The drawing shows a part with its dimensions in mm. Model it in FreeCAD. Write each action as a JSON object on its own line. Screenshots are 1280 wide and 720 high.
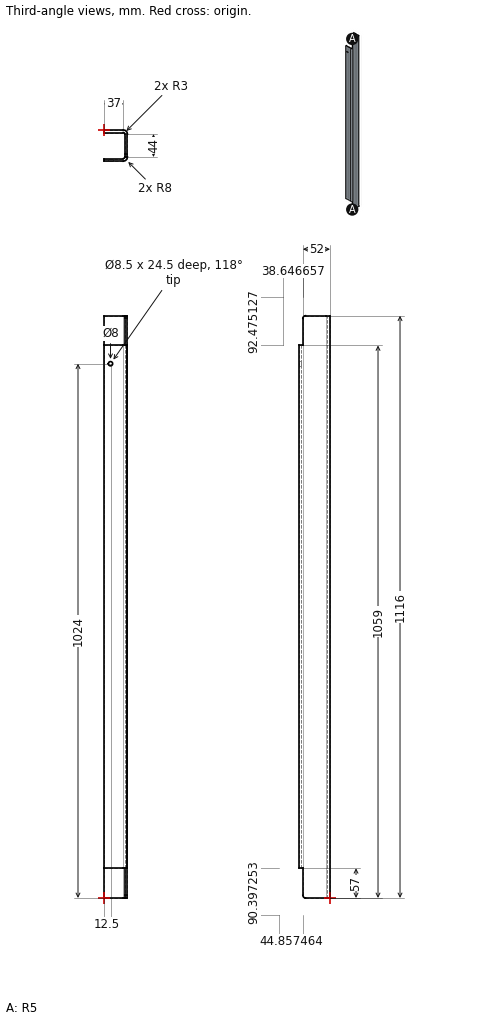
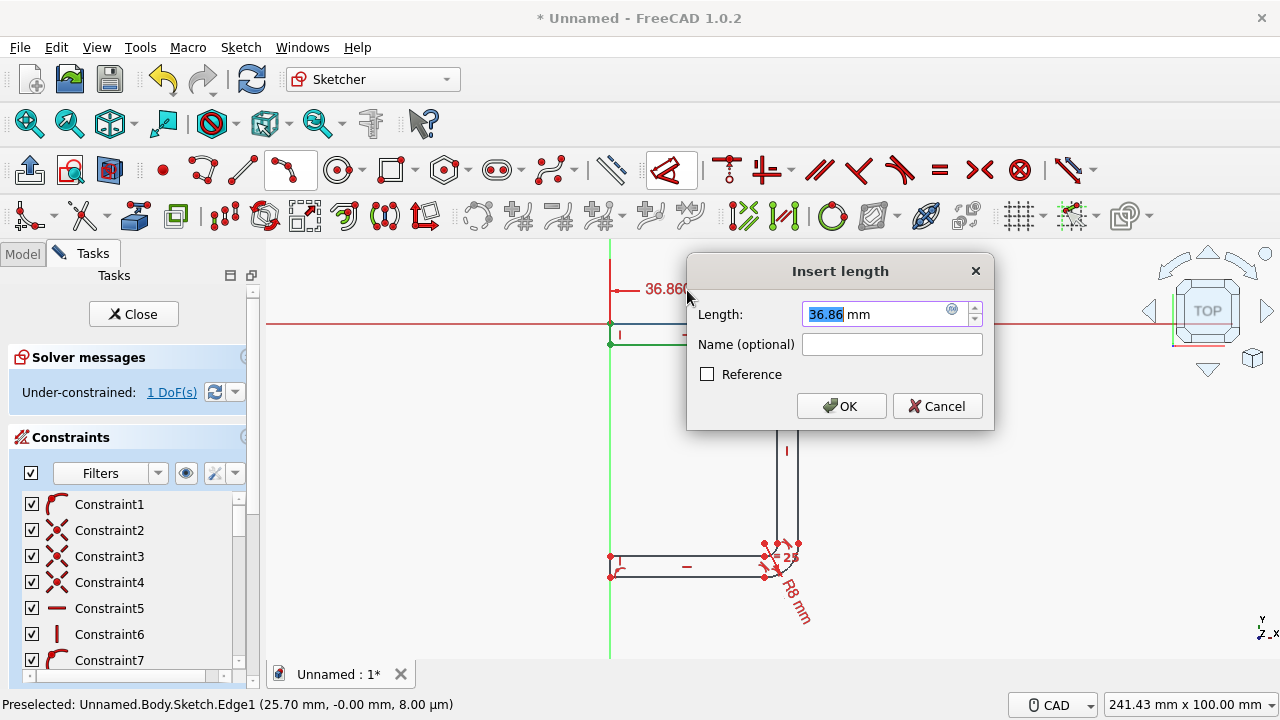
{"action": "type", "text": "37"}
{"action": "key", "text": "Return"}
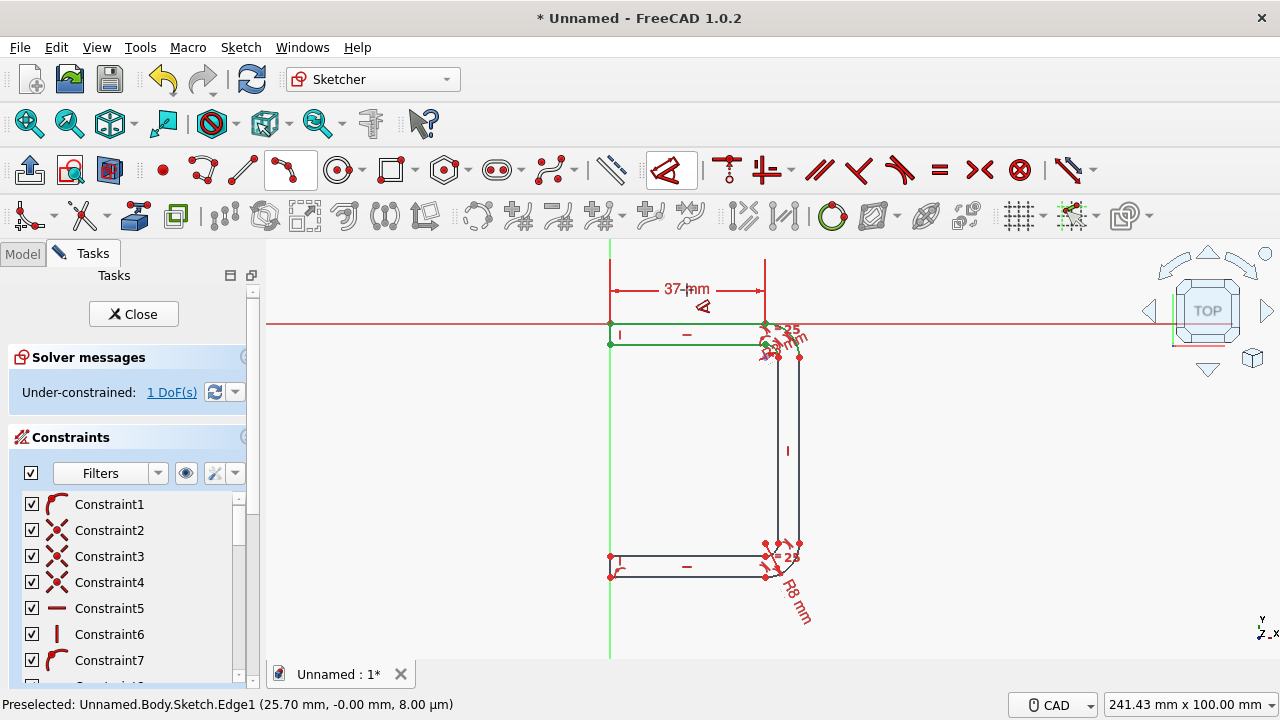
{"action": "left_click", "coordinate": [778, 413]}
{"action": "left_click", "coordinate": [812, 450]}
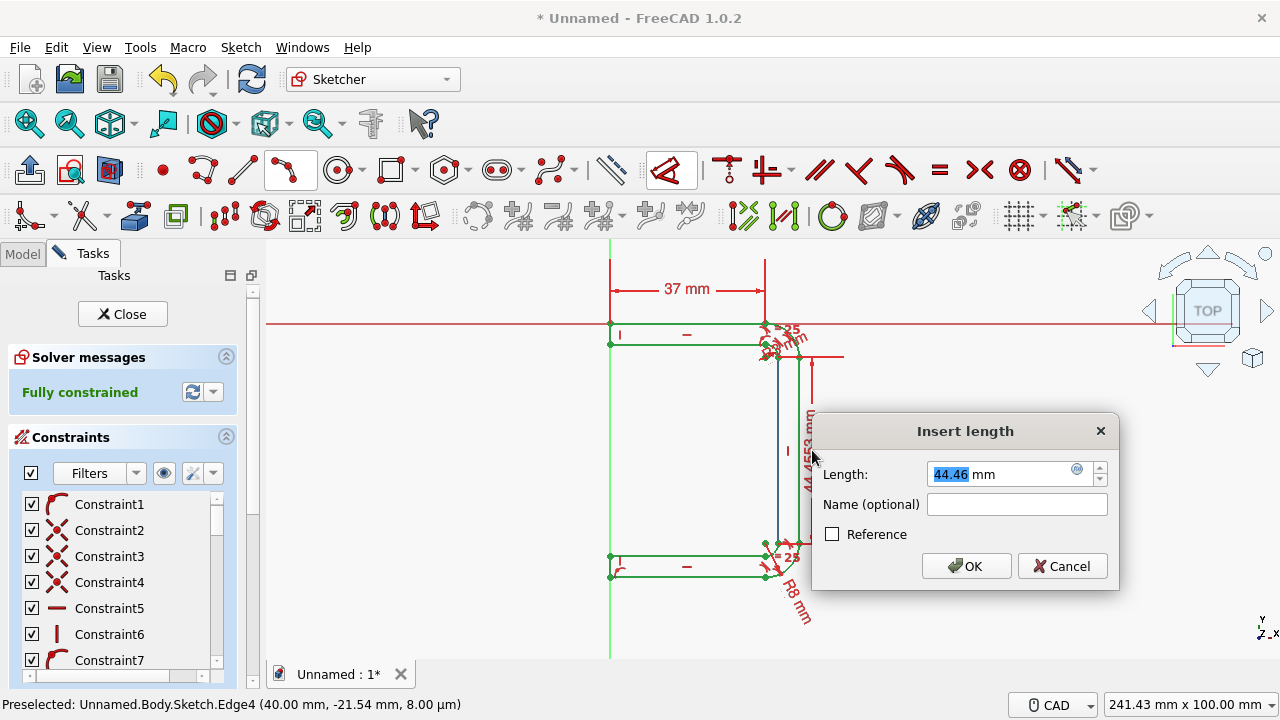
{"action": "type", "text": "44"}
{"action": "key", "text": "Return"}
{"action": "key", "text": "Escape"}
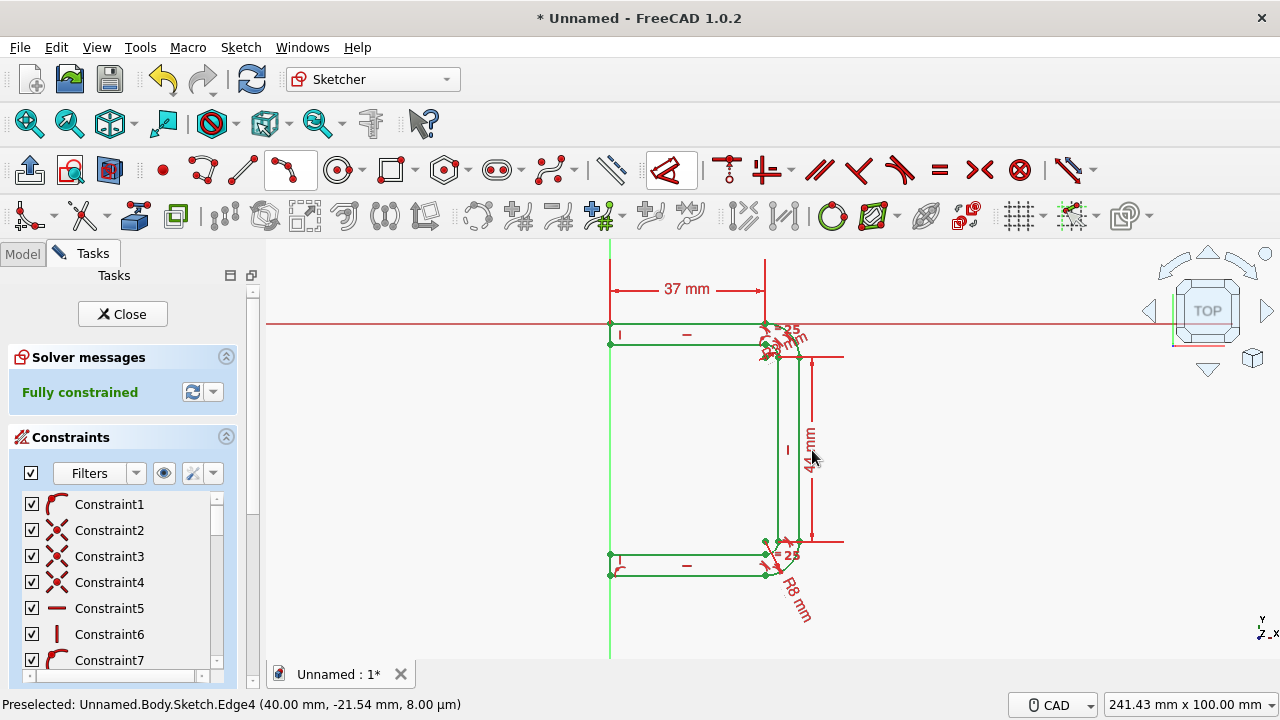
{"action": "left_click", "coordinate": [123, 314]}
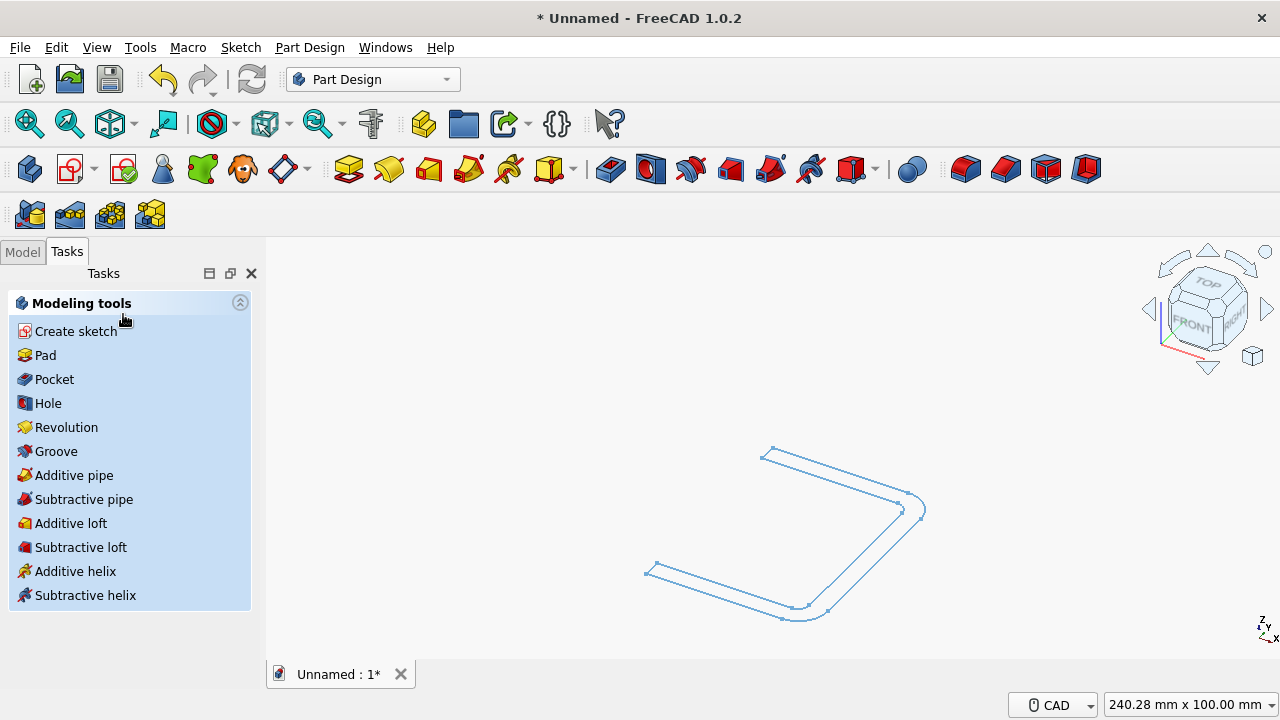
{"action": "left_click", "coordinate": [350, 170]}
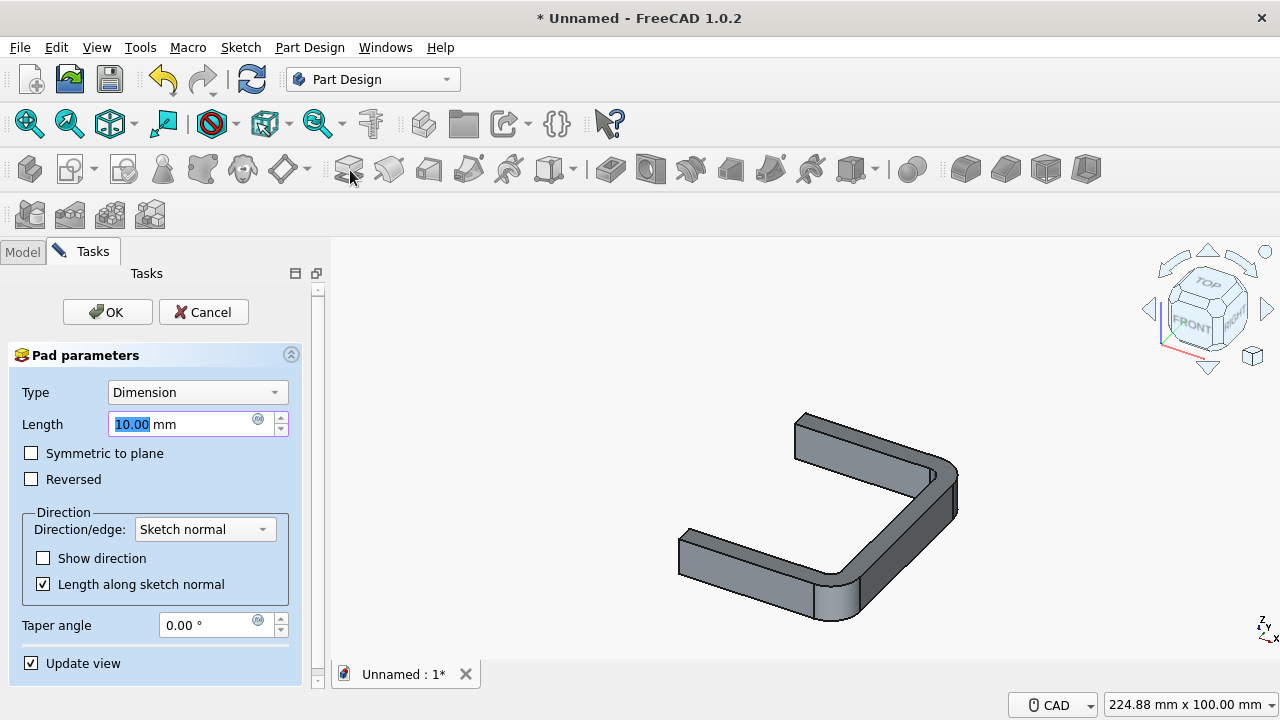
{"action": "type", "text": "1116"}
{"action": "key", "text": "Tab"}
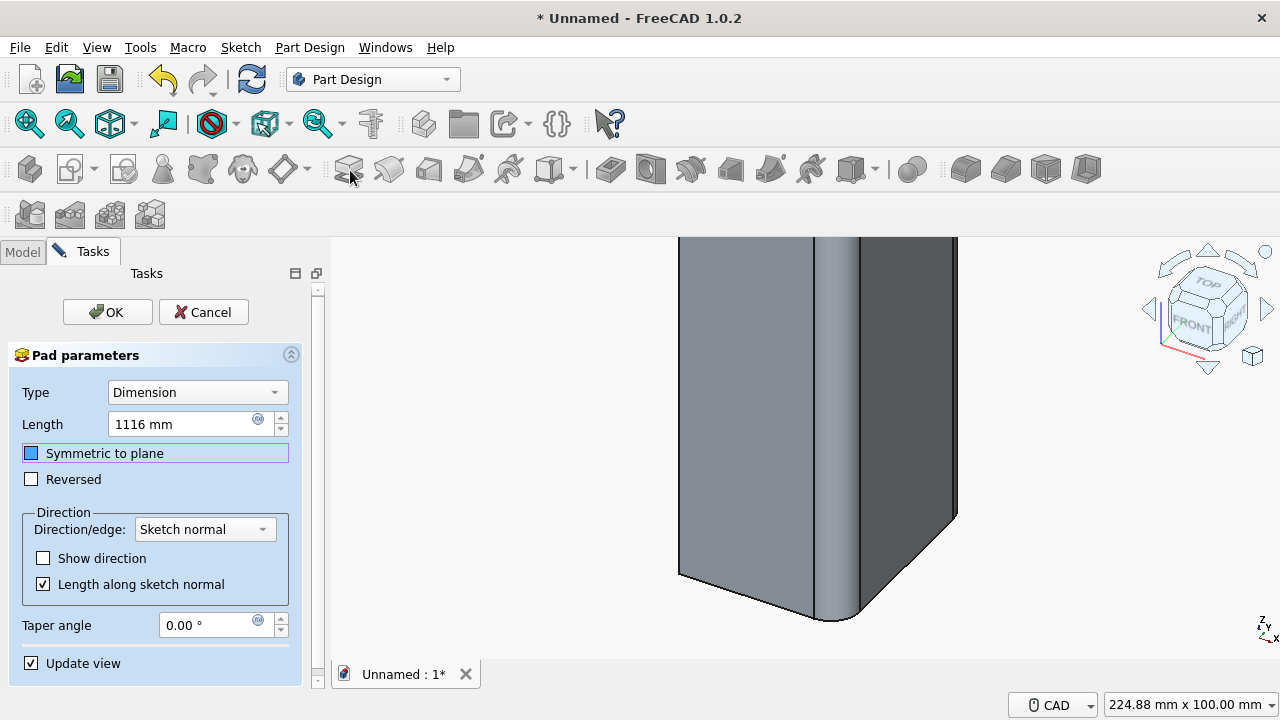
{"action": "left_click", "coordinate": [108, 312]}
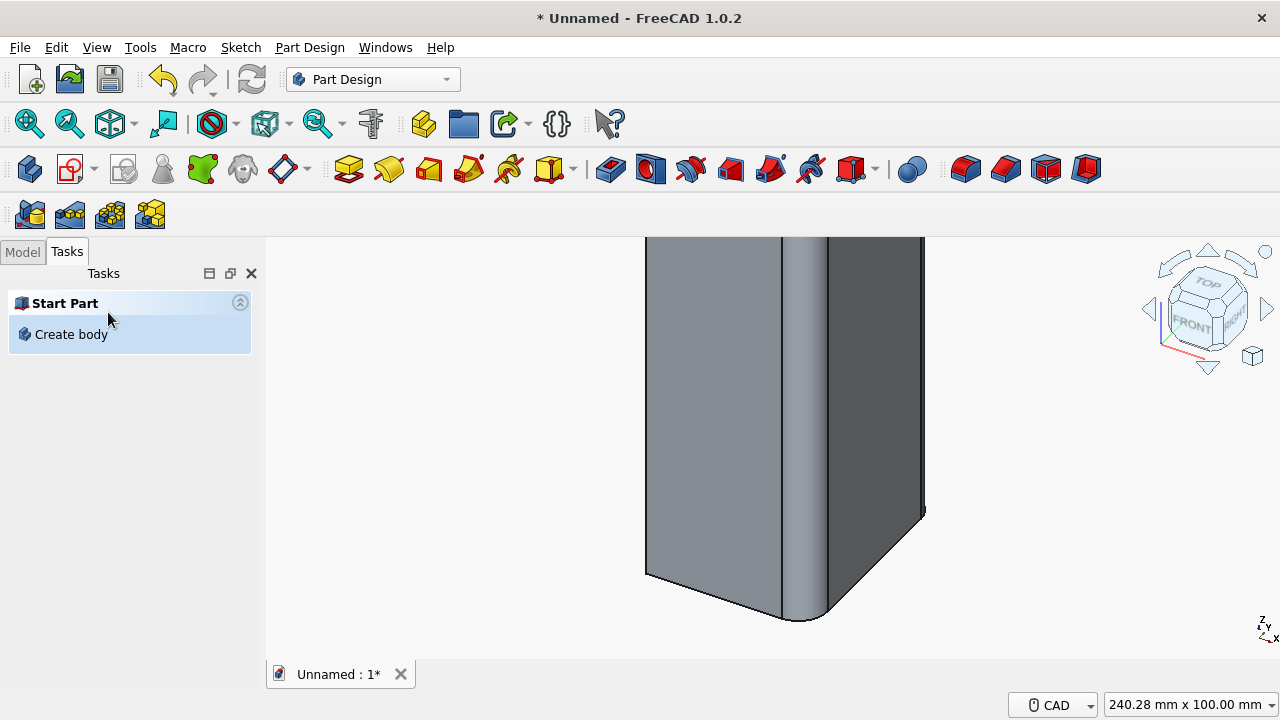
{"action": "key", "text": "v f"}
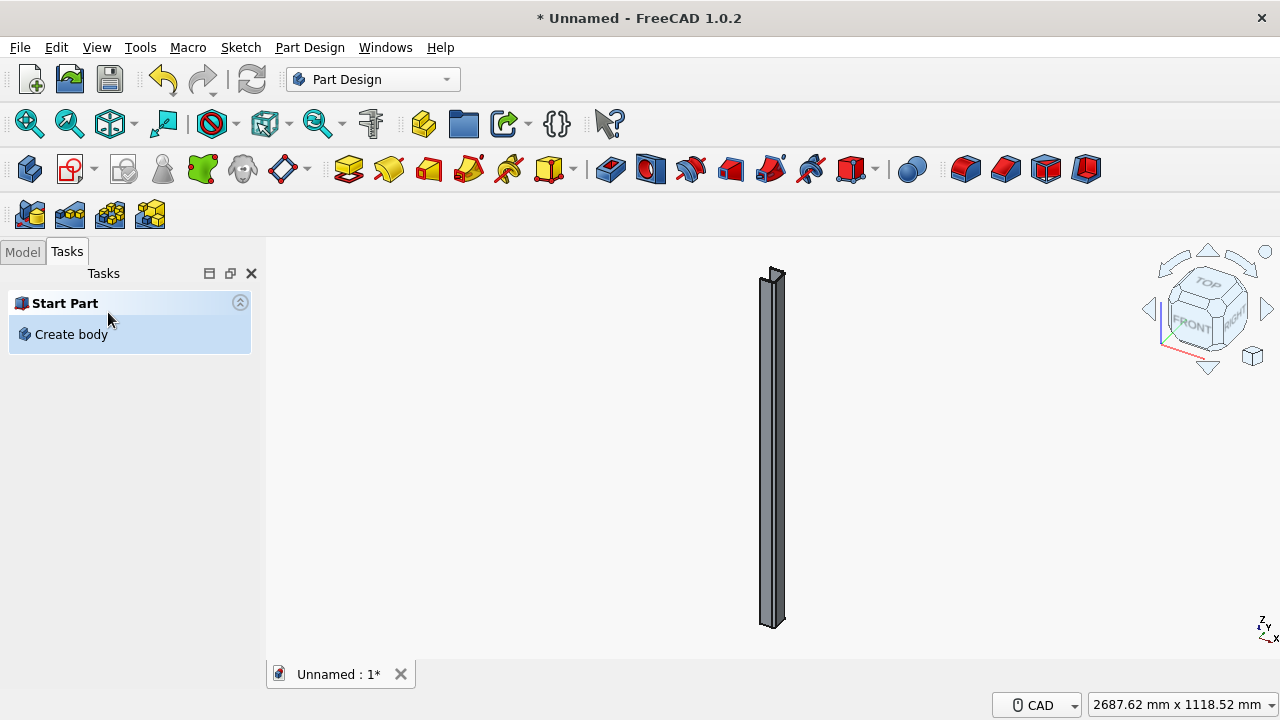
{"action": "key", "text": "6"}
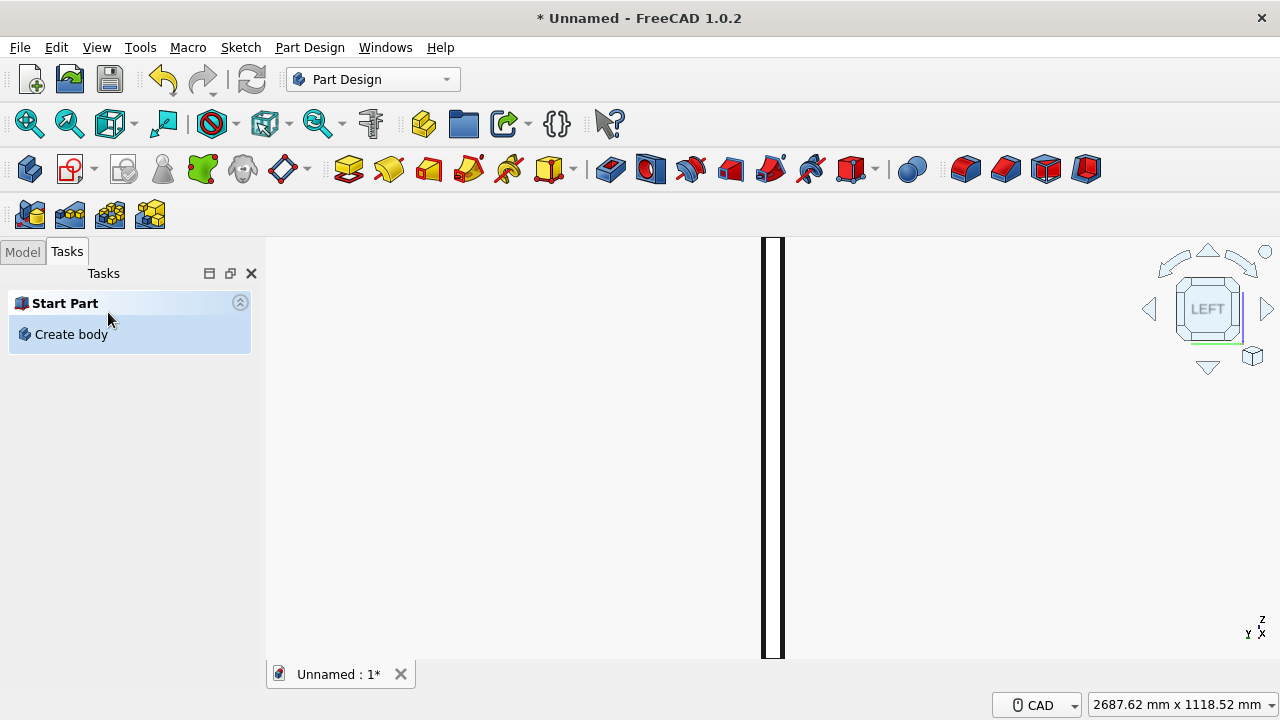
{"action": "key", "text": "v f"}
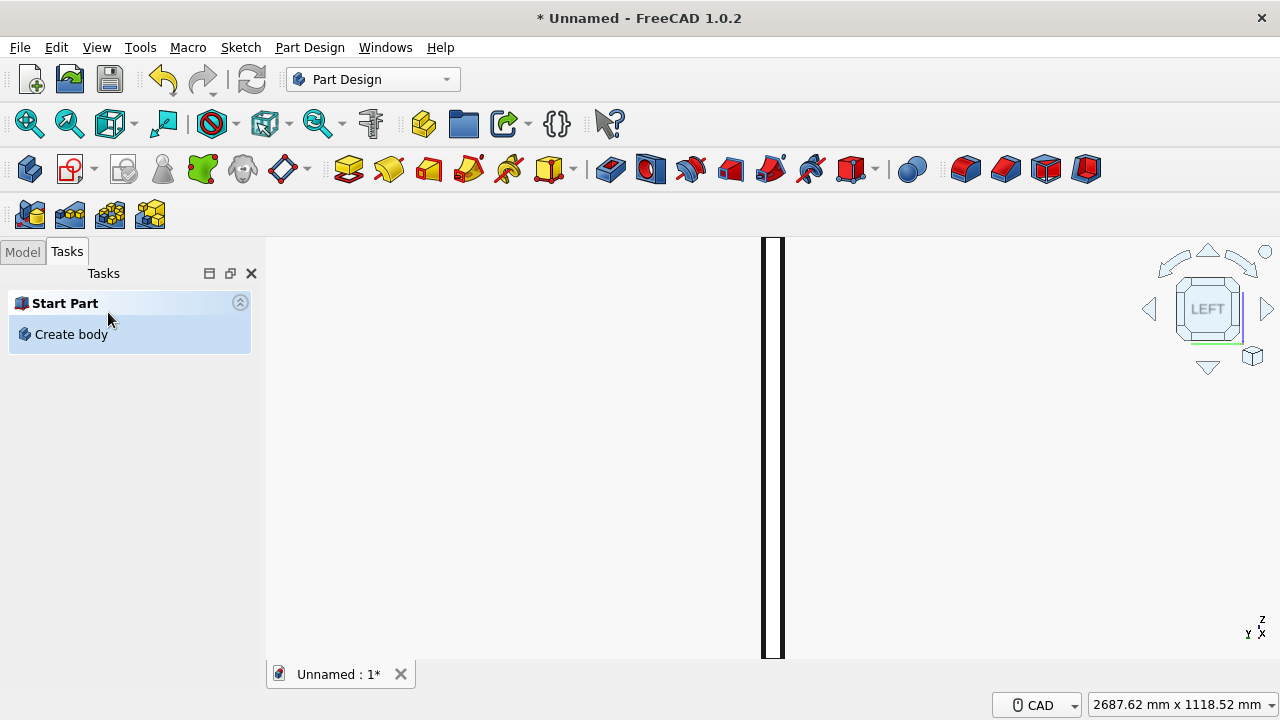
{"action": "scroll", "coordinate": [763, 267], "scroll_direction": "up", "scroll_amount": 13}